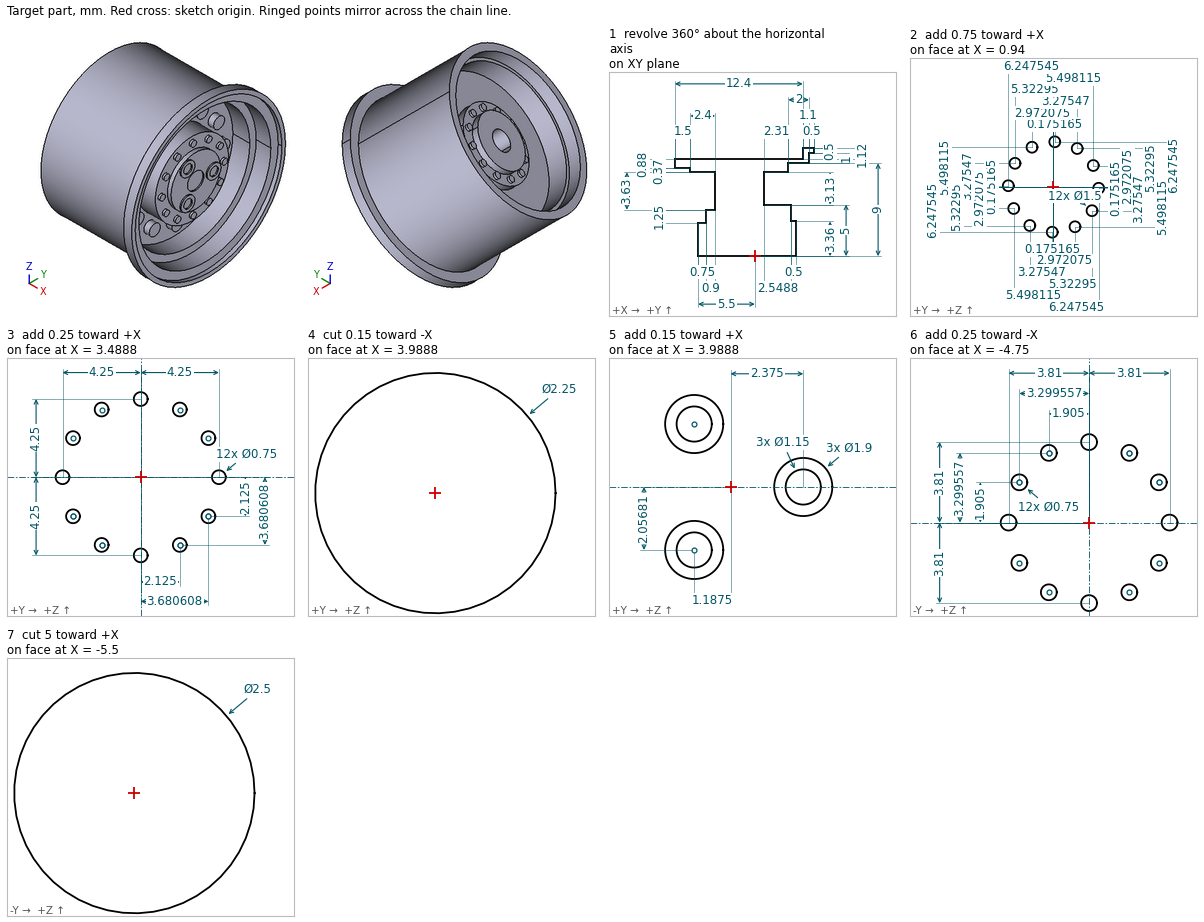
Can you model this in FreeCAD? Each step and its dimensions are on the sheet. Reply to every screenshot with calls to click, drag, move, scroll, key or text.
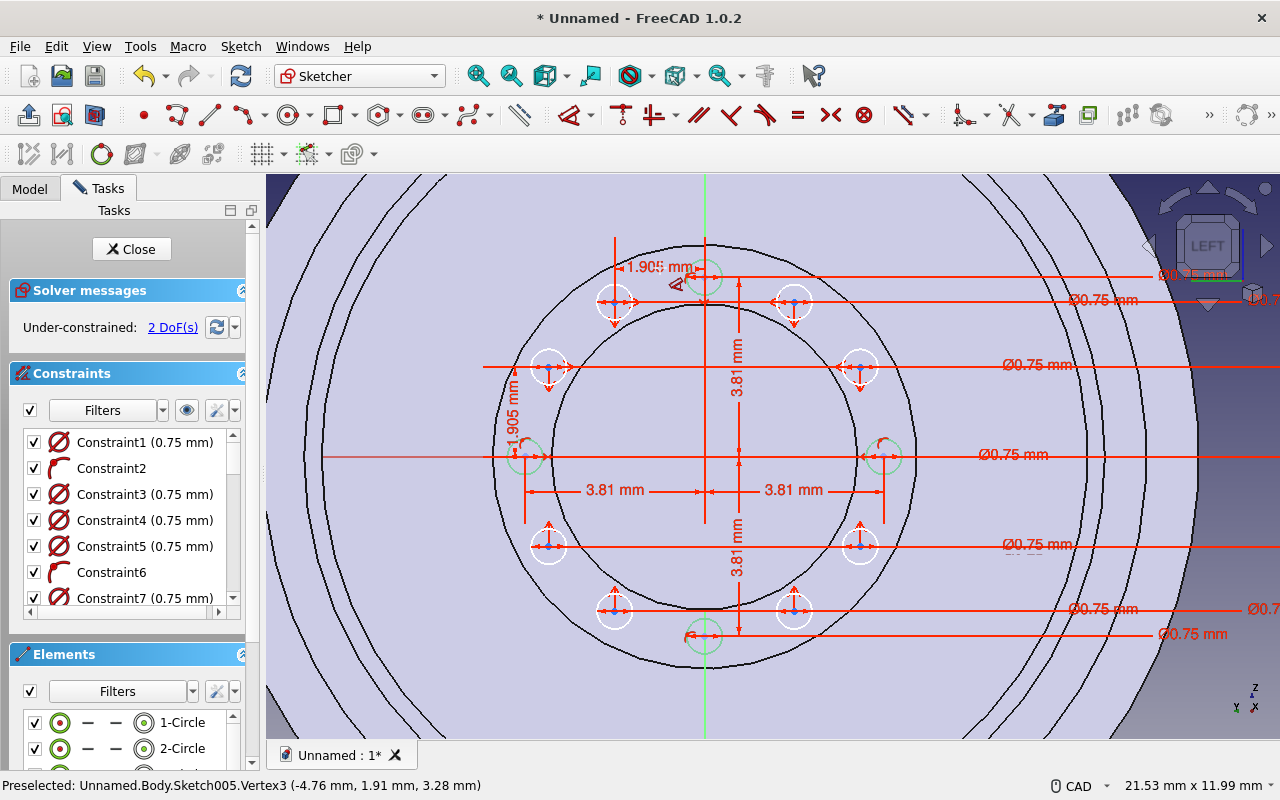
click(549, 367)
click(627, 333)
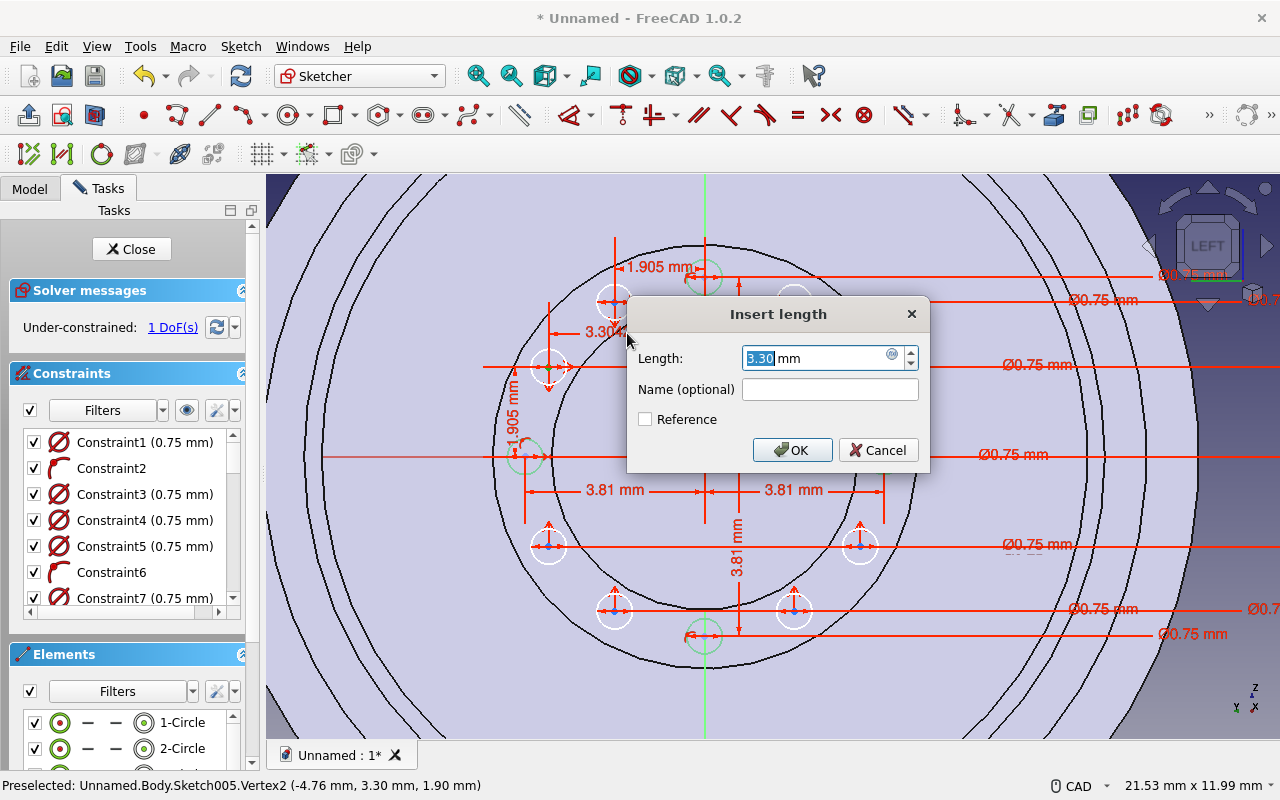
text(3.299557)
key(Return)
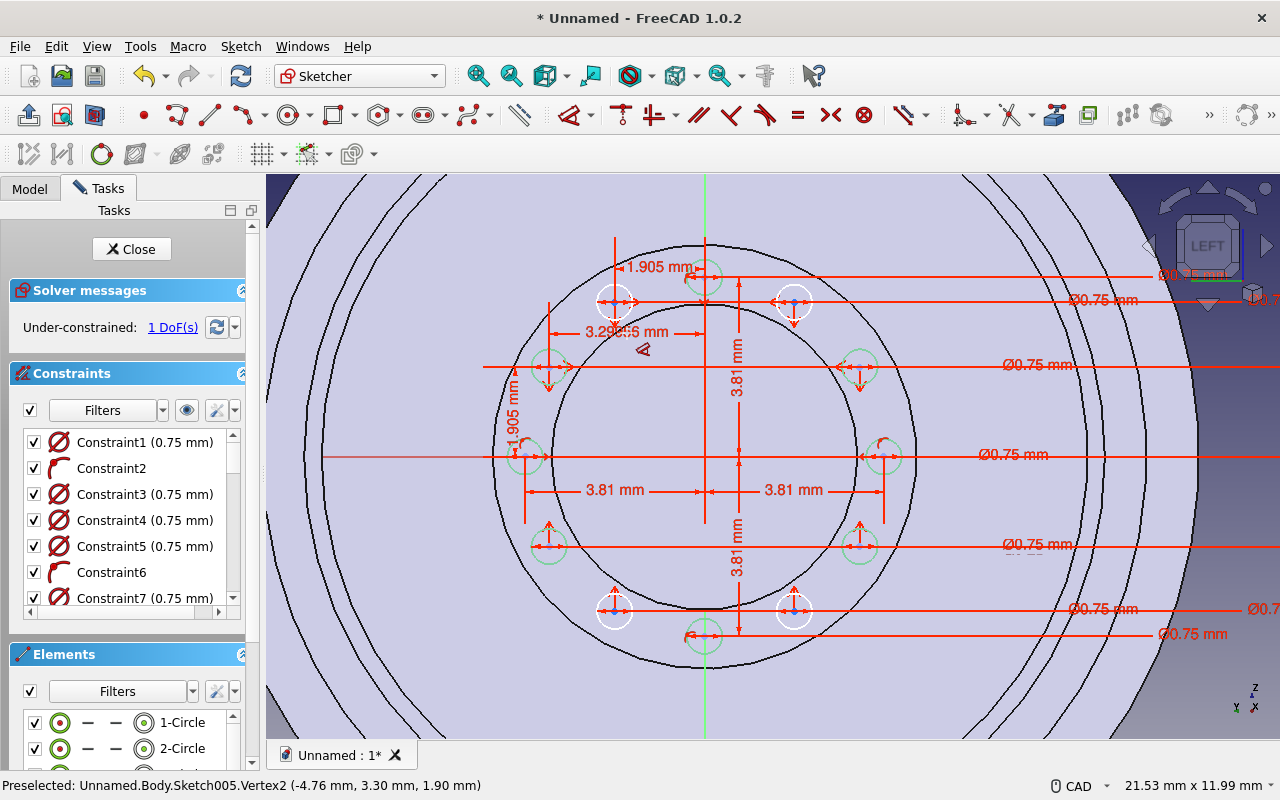
click(615, 302)
click(581, 380)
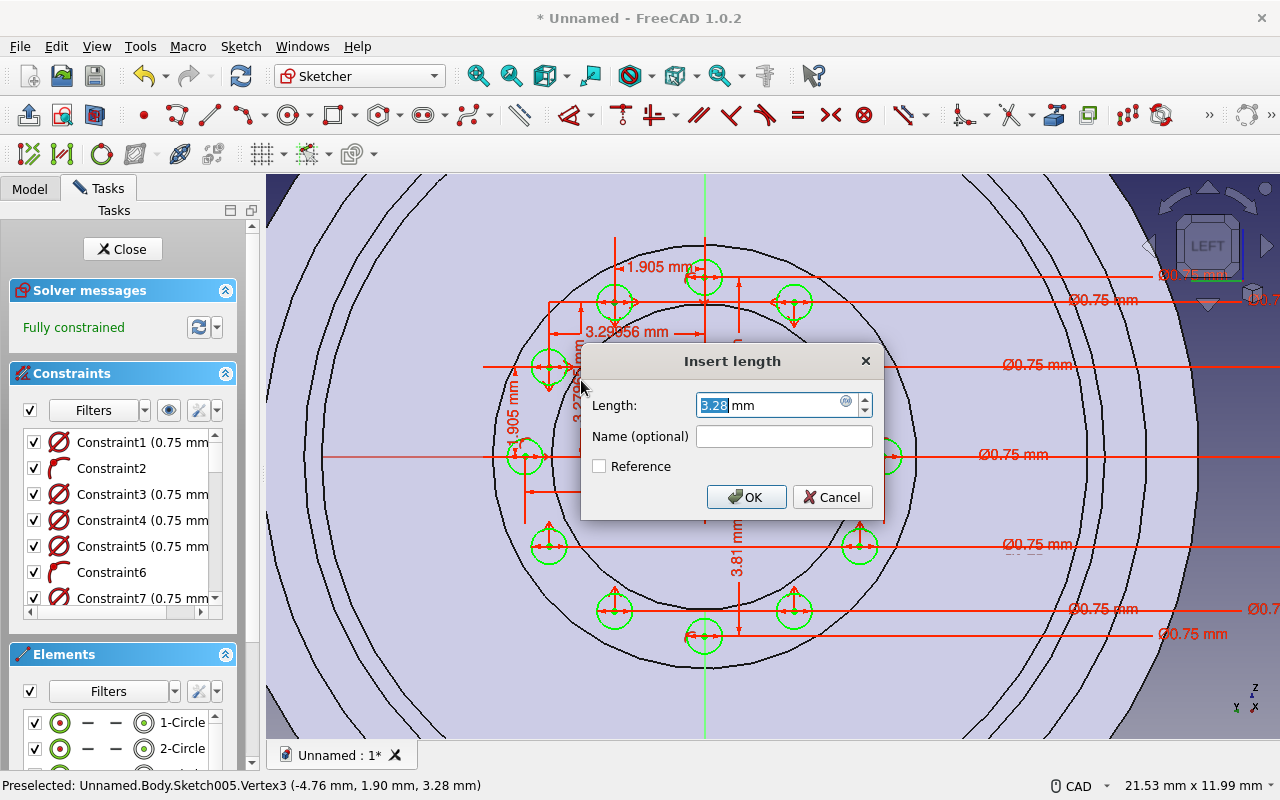
text(3.299557)
key(Return)
key(Escape)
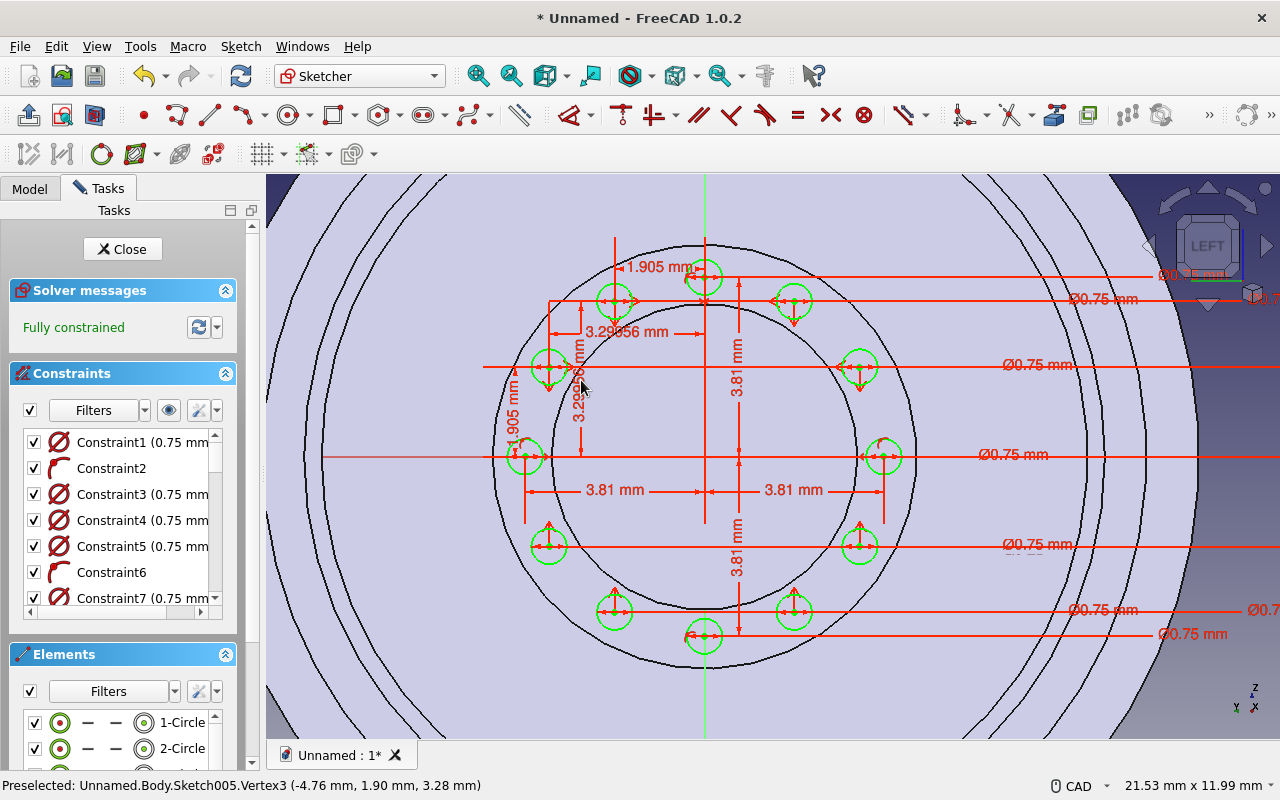
click(123, 249)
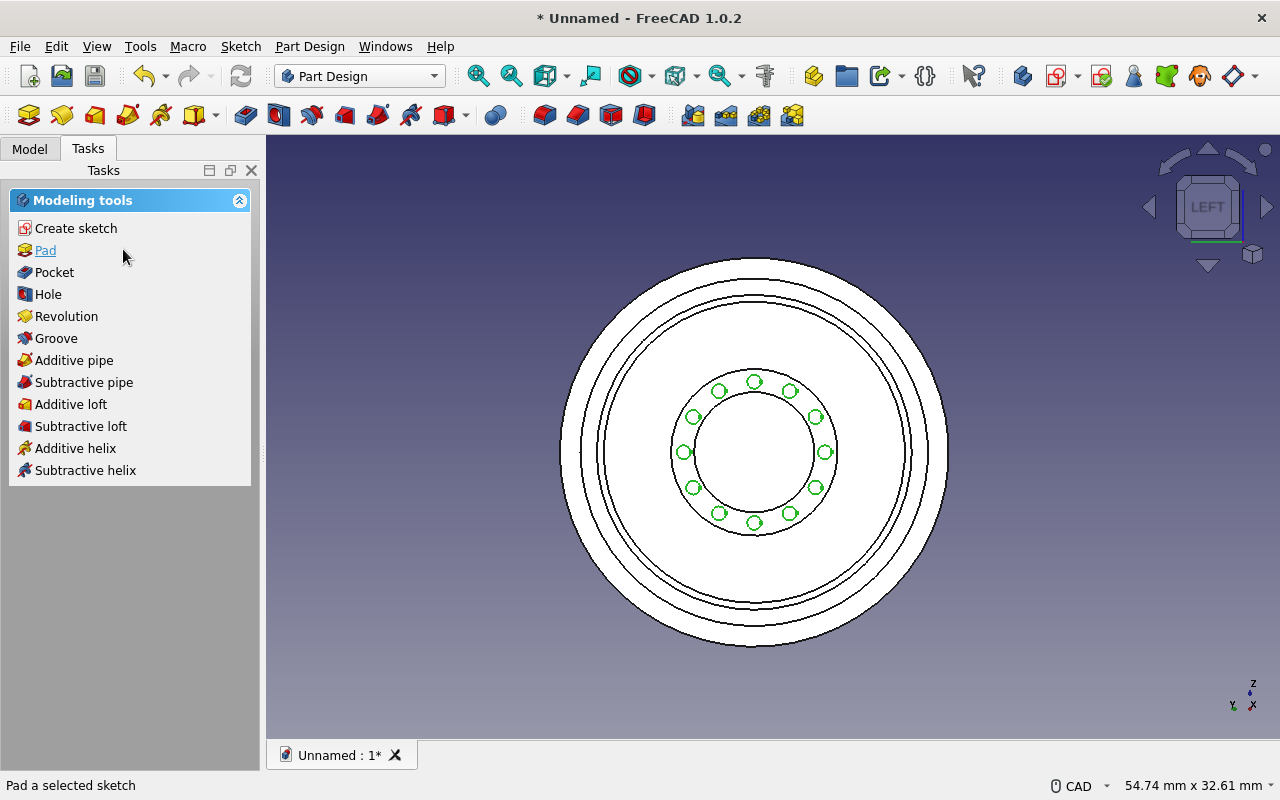
click(29, 116)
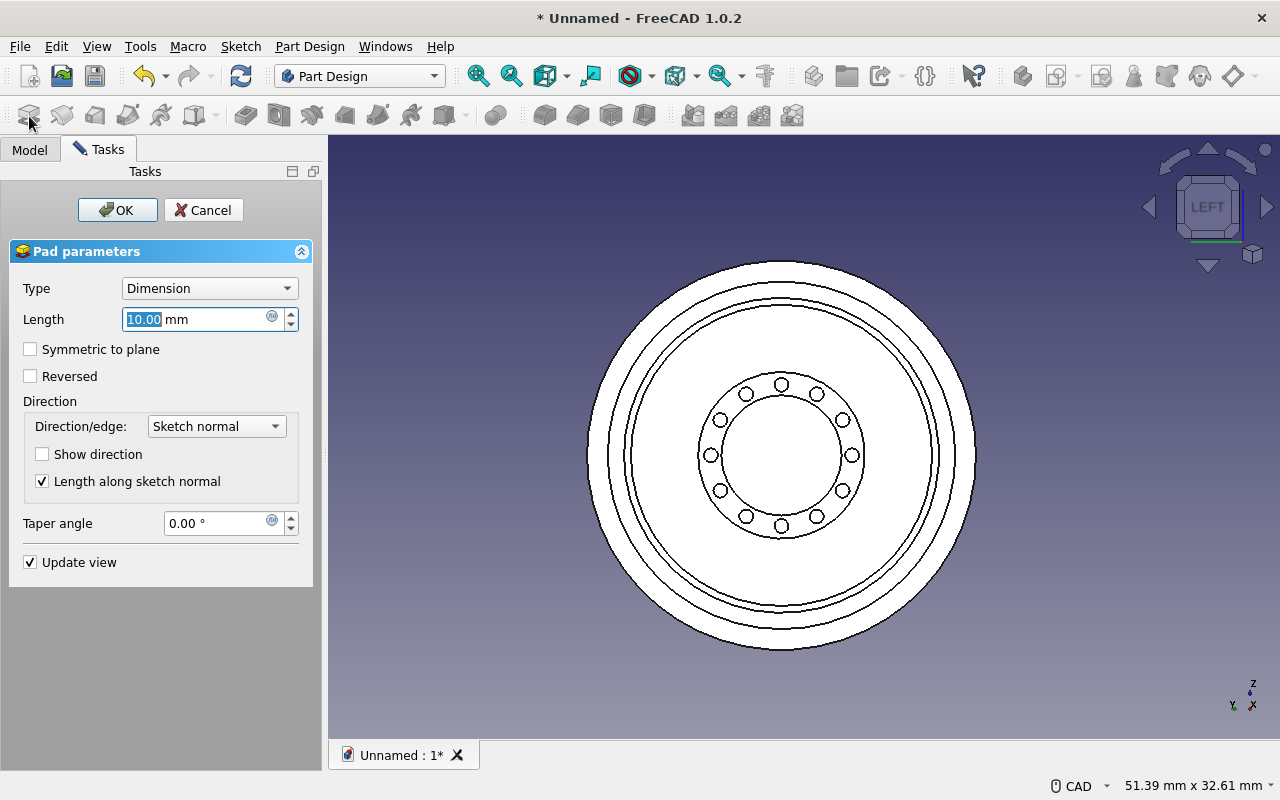
text(0.25)
key(Tab)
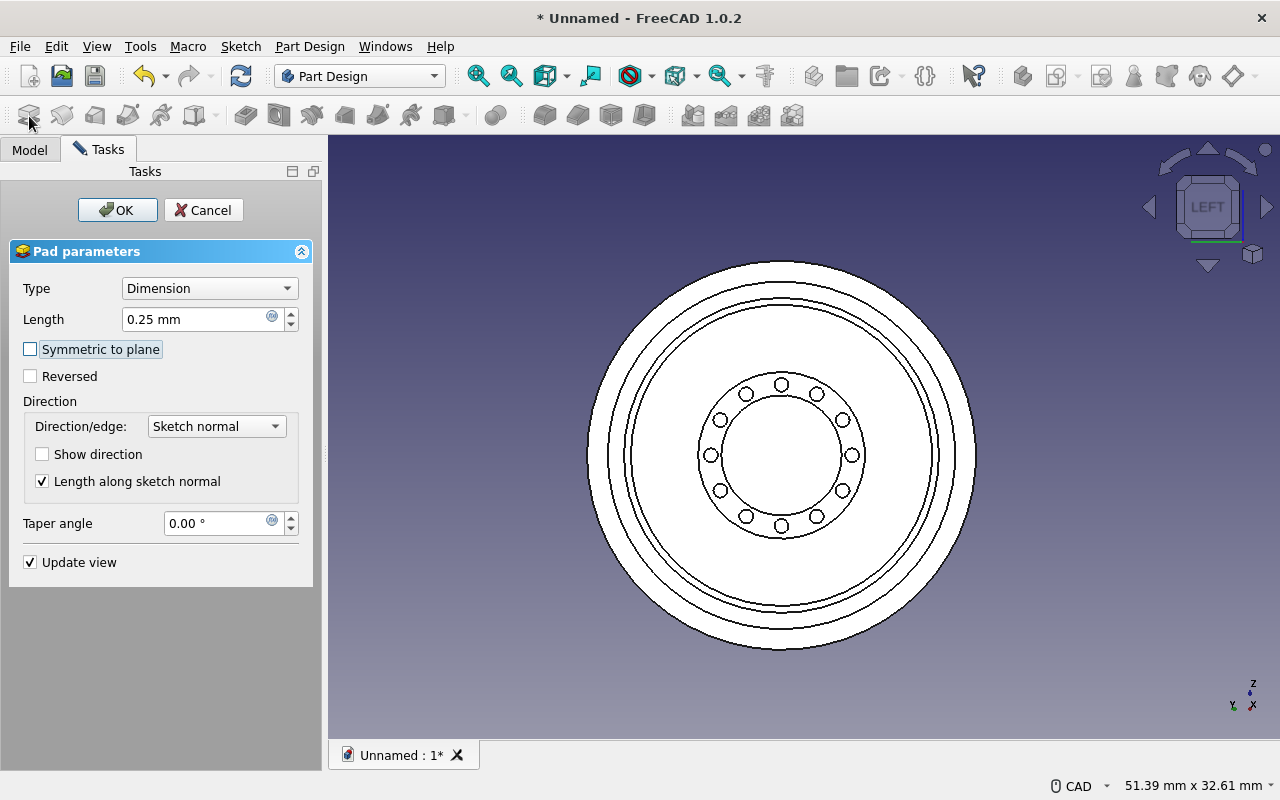
click(118, 210)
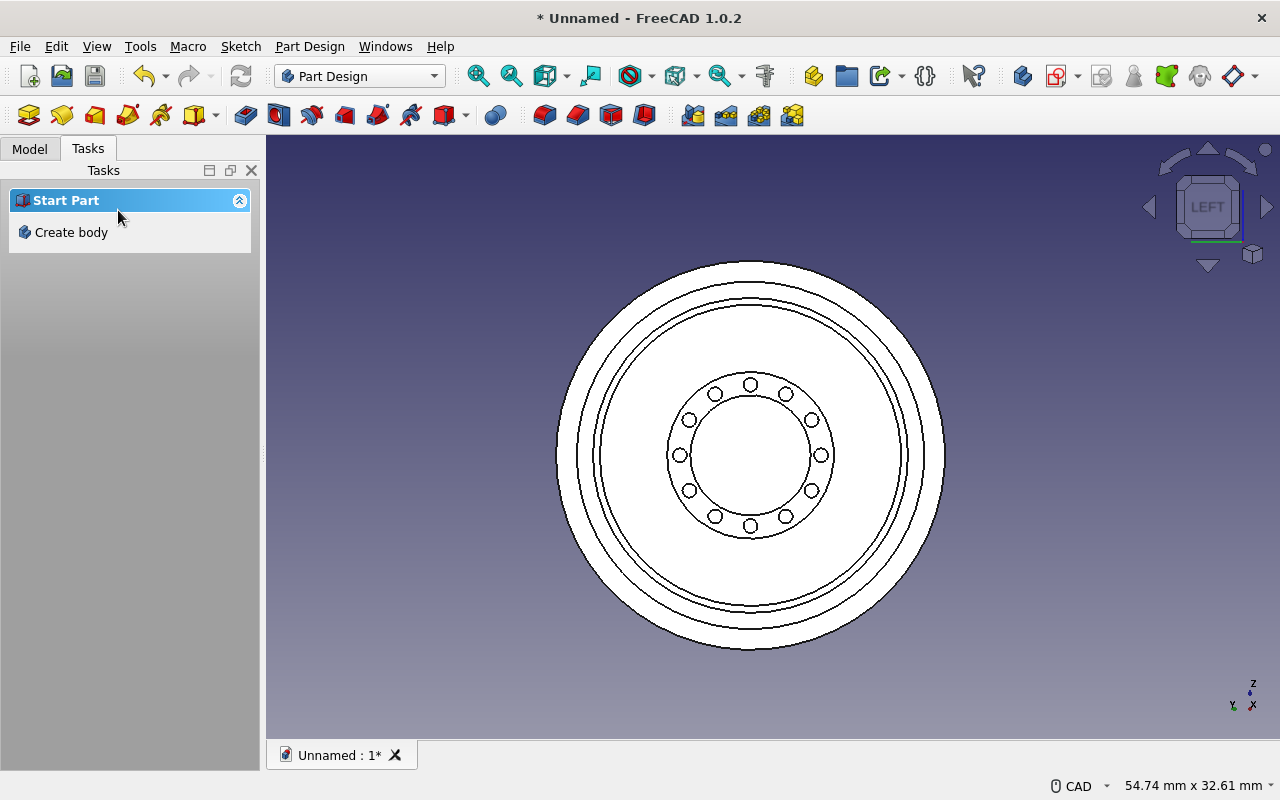
click(750, 454)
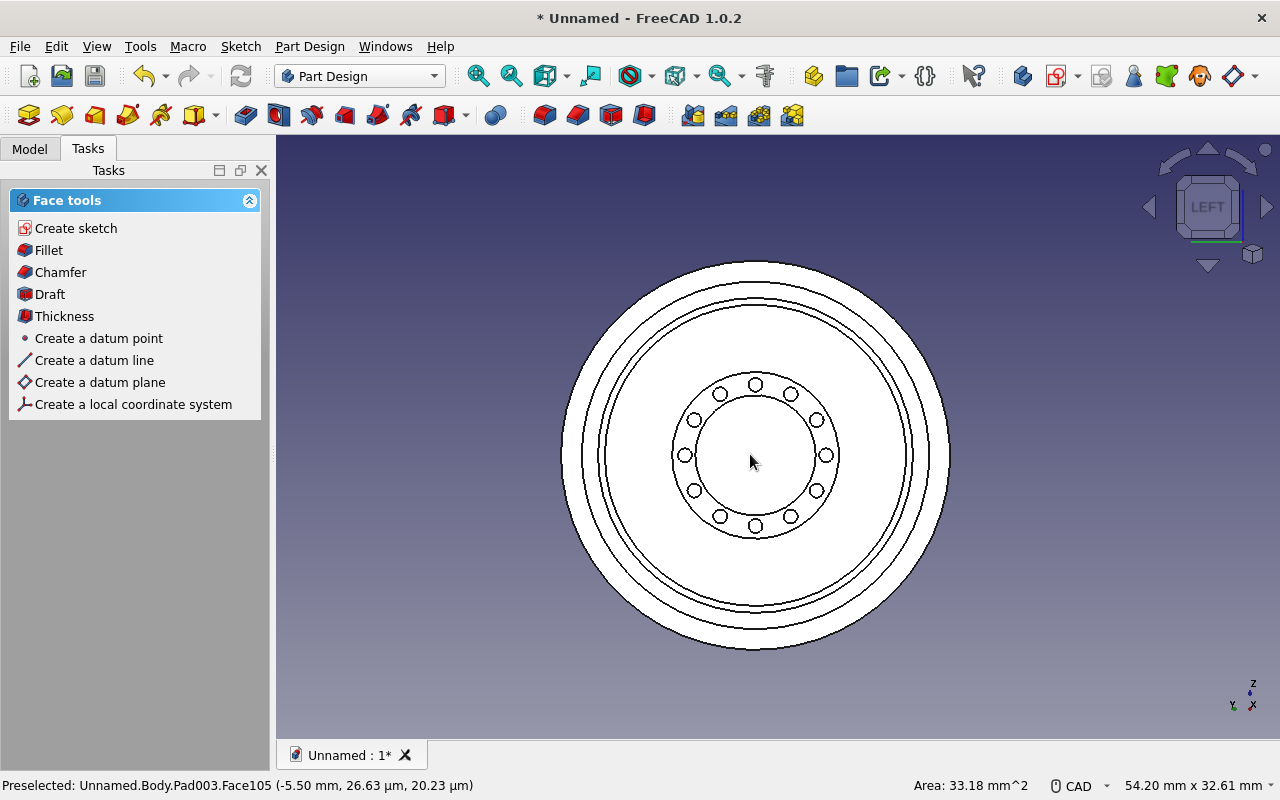
click(1056, 76)